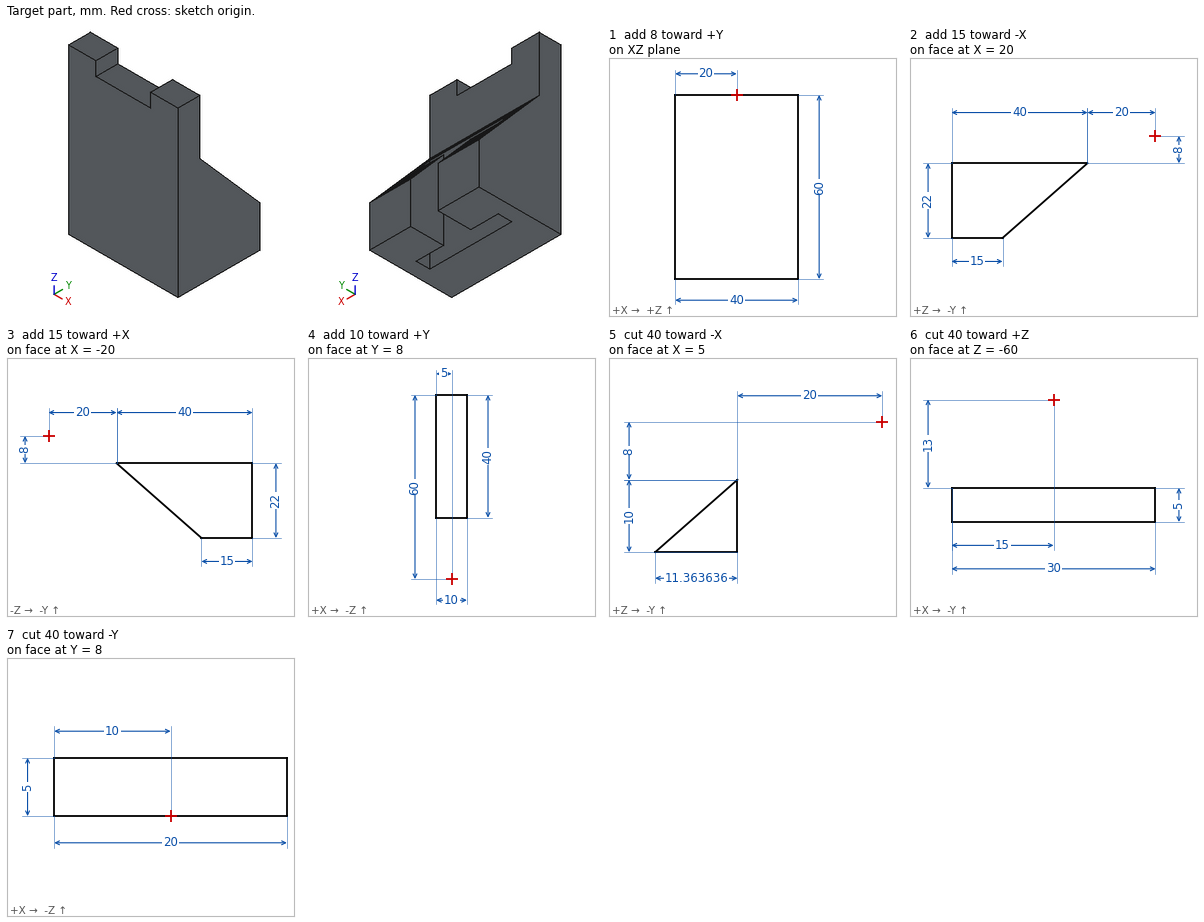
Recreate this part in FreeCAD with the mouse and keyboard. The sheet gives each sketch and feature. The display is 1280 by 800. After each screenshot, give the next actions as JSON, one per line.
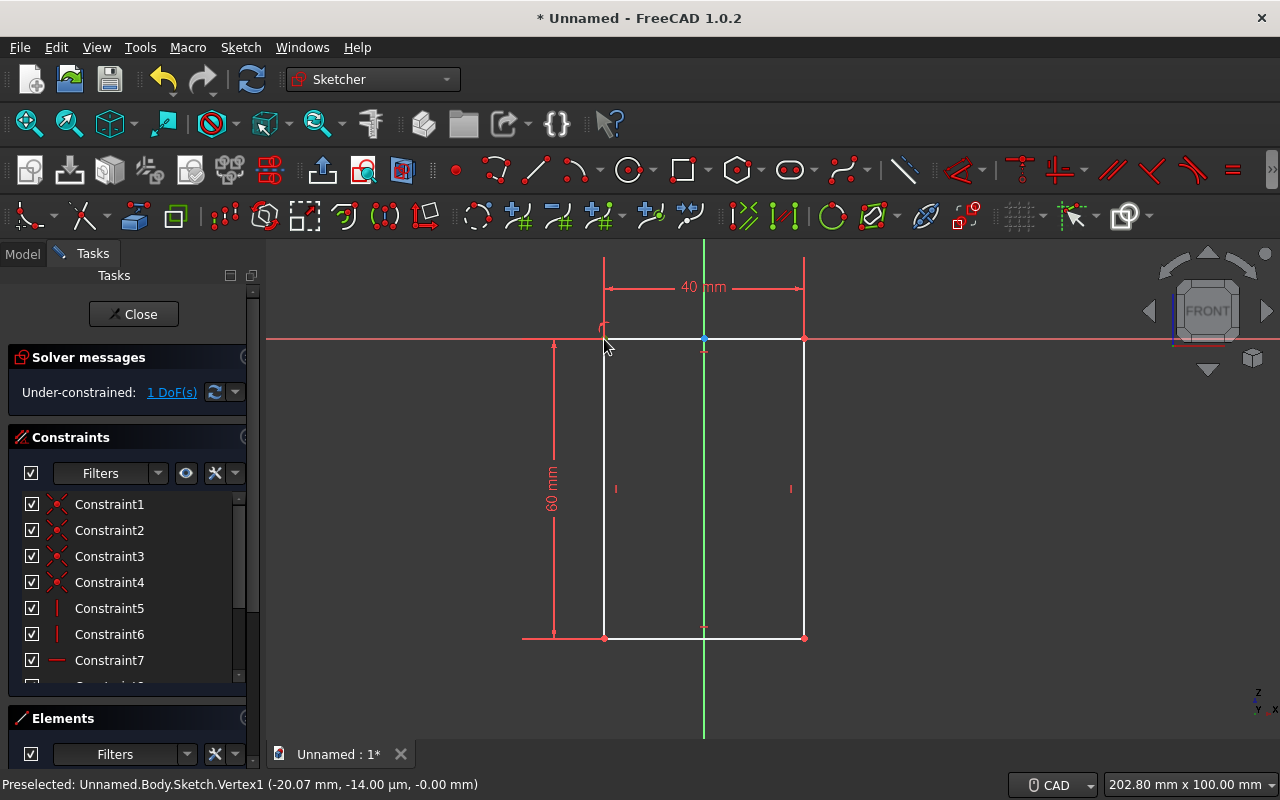
{"action": "key", "text": "l"}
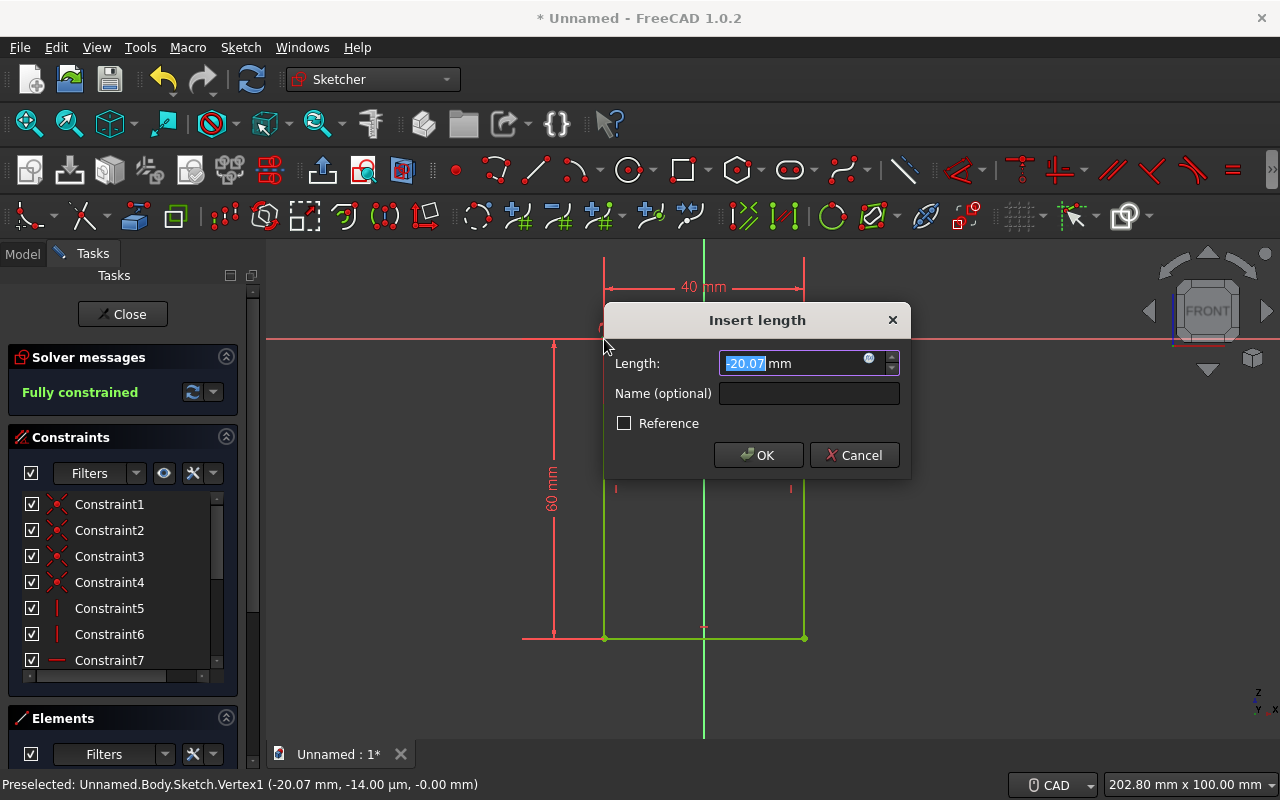
{"action": "type", "text": "-20"}
{"action": "key", "text": "Return"}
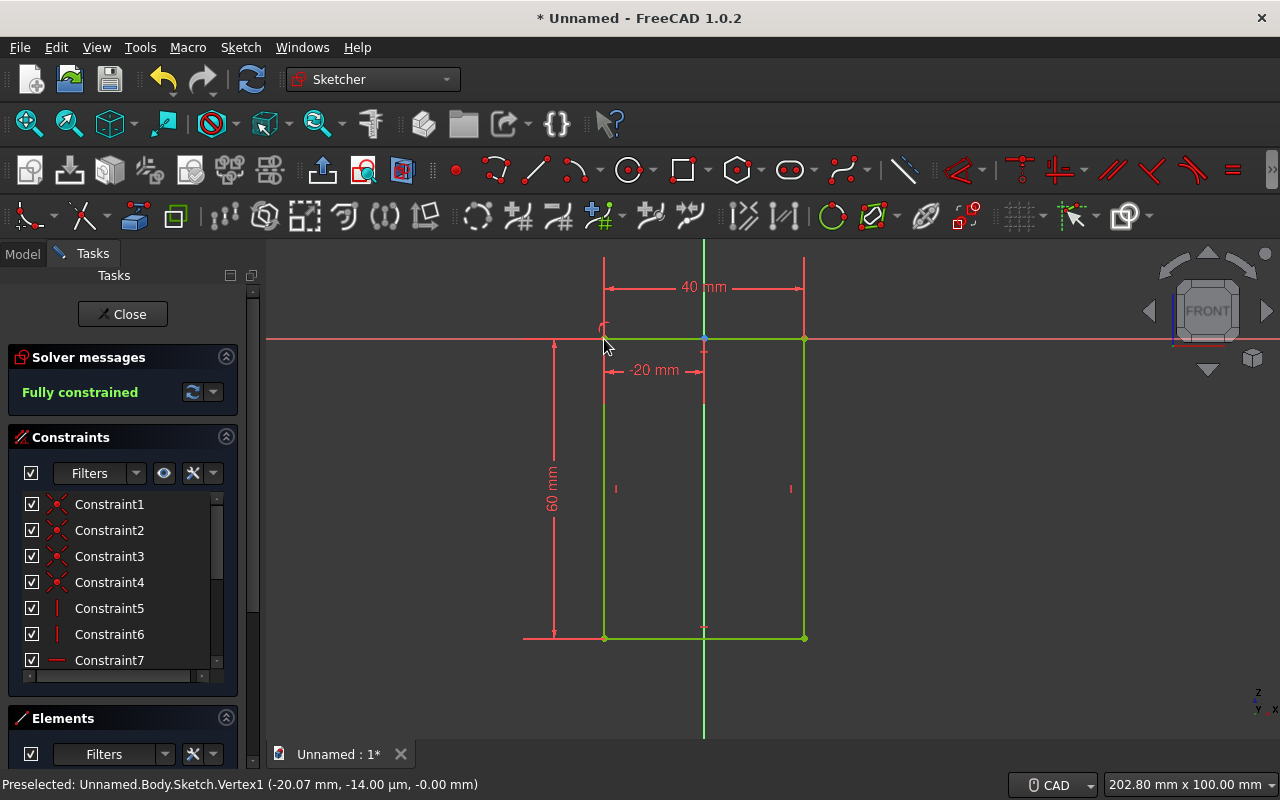
{"action": "left_click", "coordinate": [123, 314]}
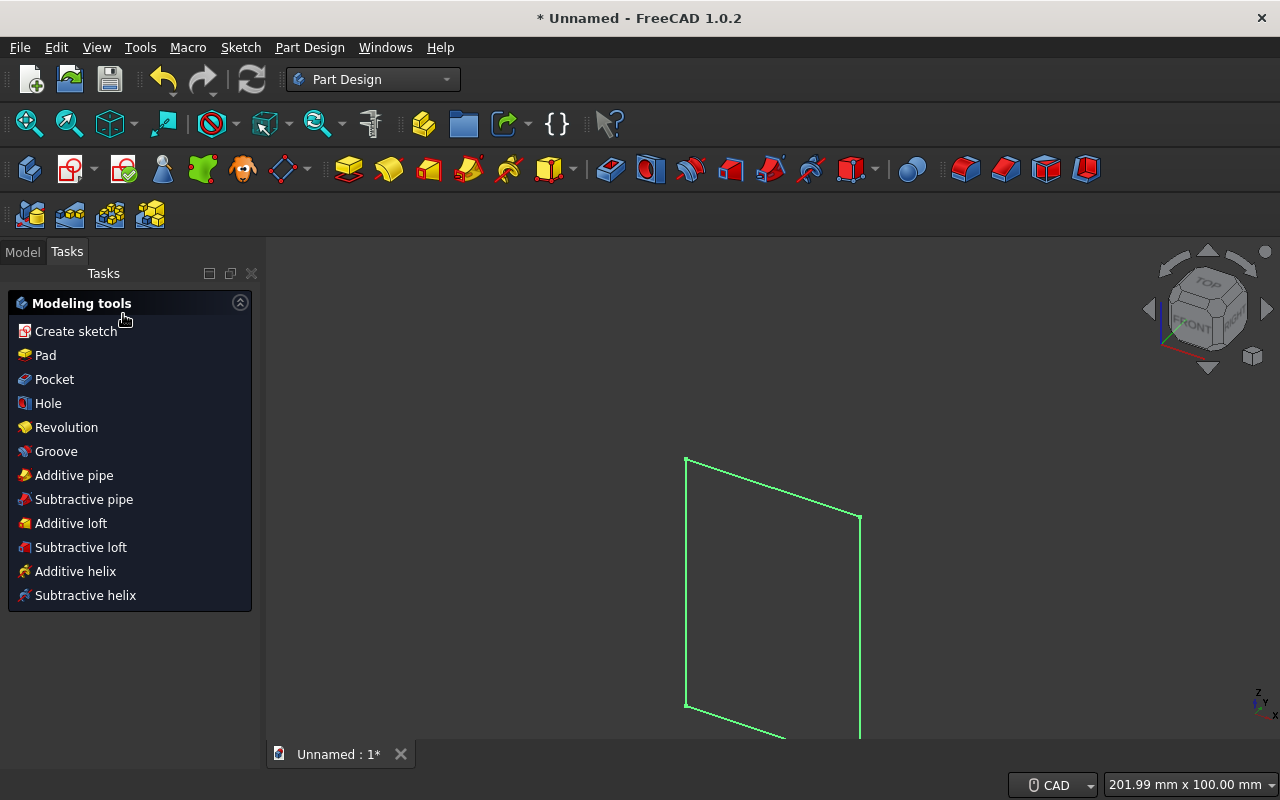
{"action": "left_click", "coordinate": [350, 170]}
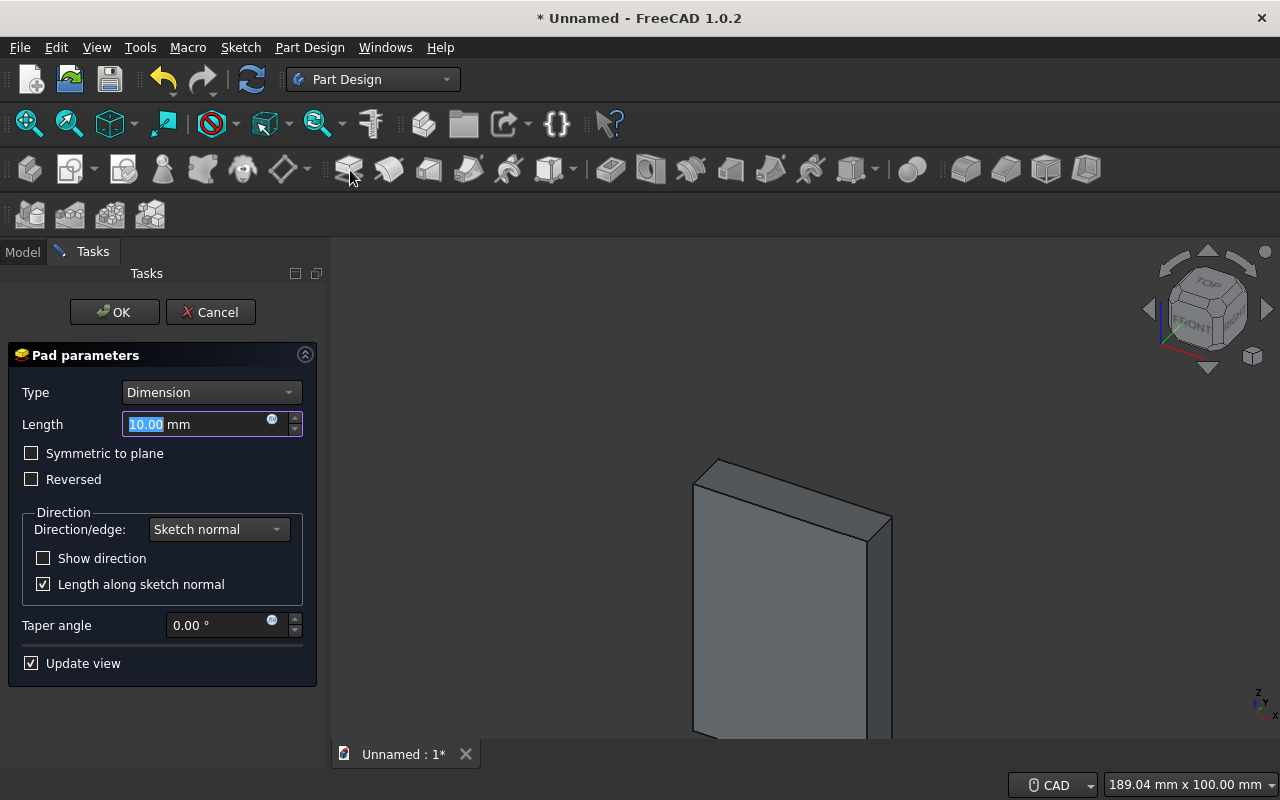
{"action": "type", "text": "8"}
{"action": "key", "text": "Tab"}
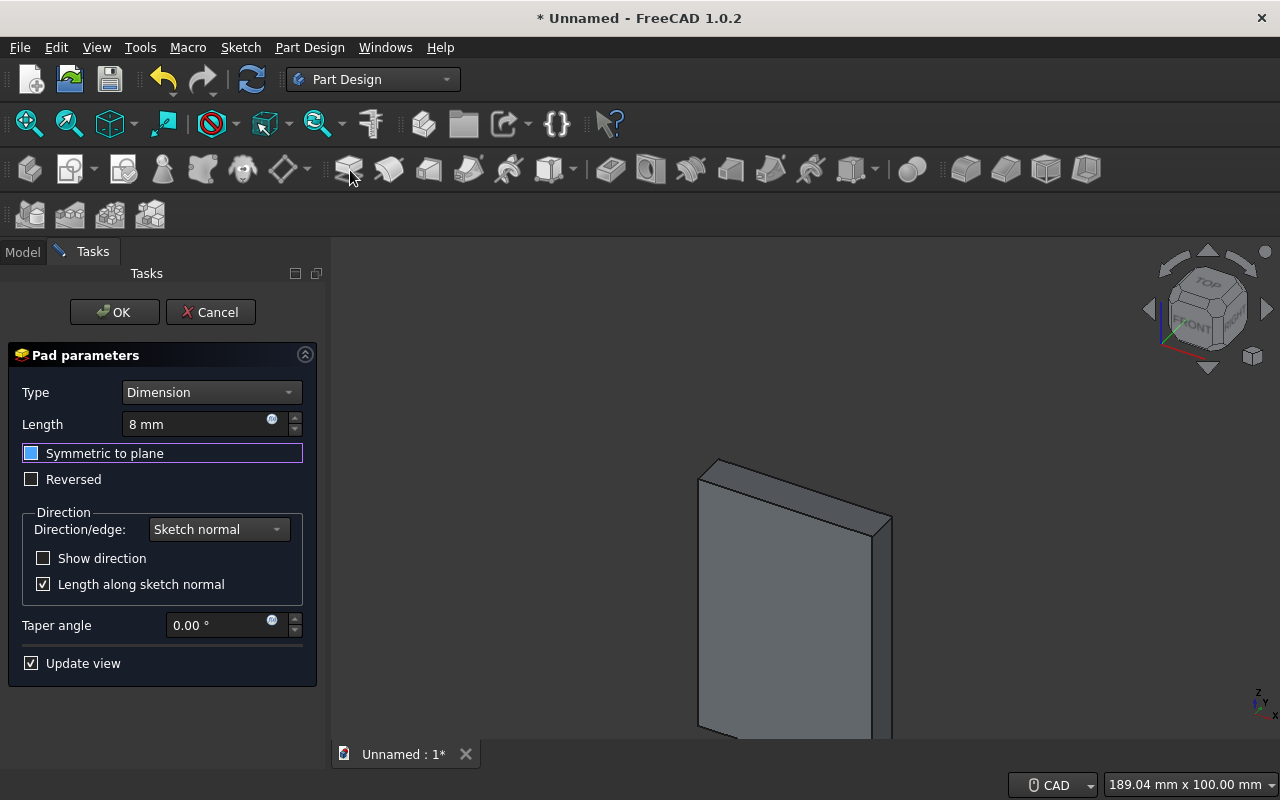
{"action": "left_click", "coordinate": [30, 479]}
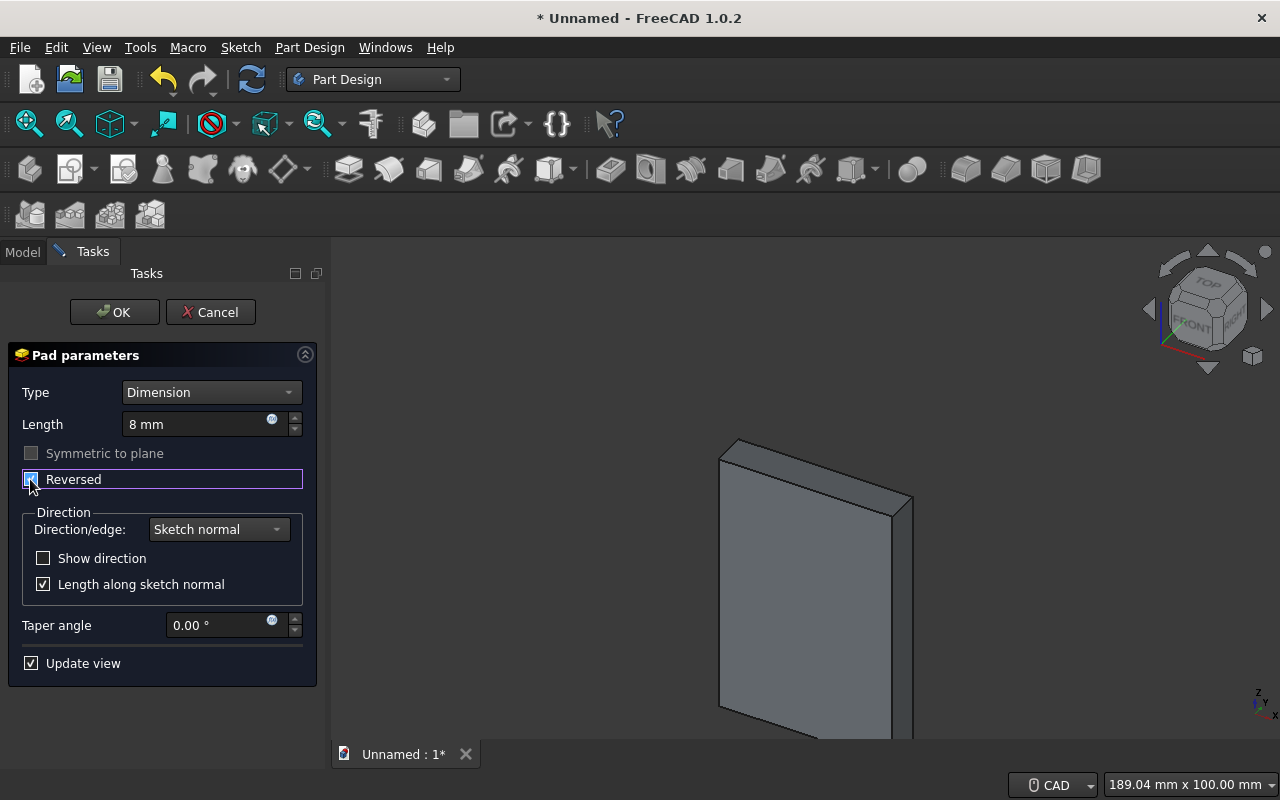
{"action": "left_click", "coordinate": [115, 312]}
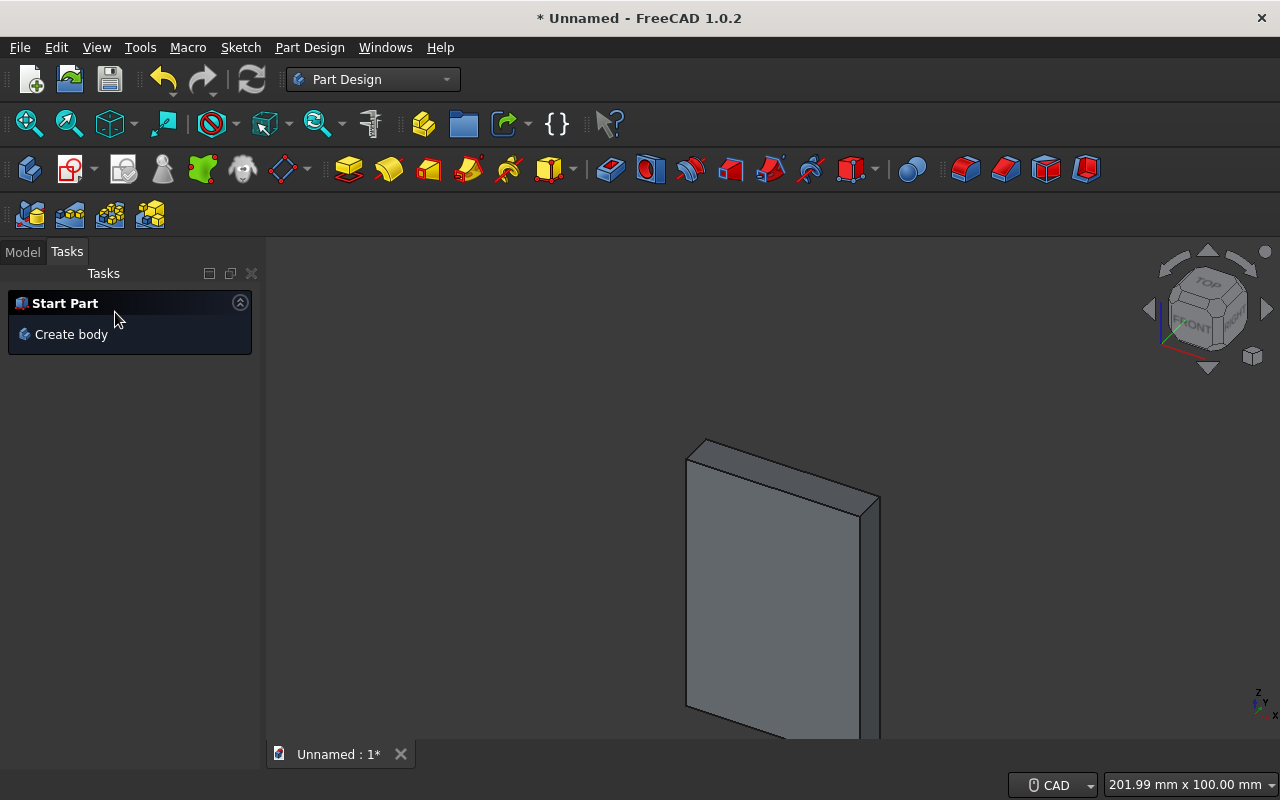
{"action": "left_click", "coordinate": [30, 124]}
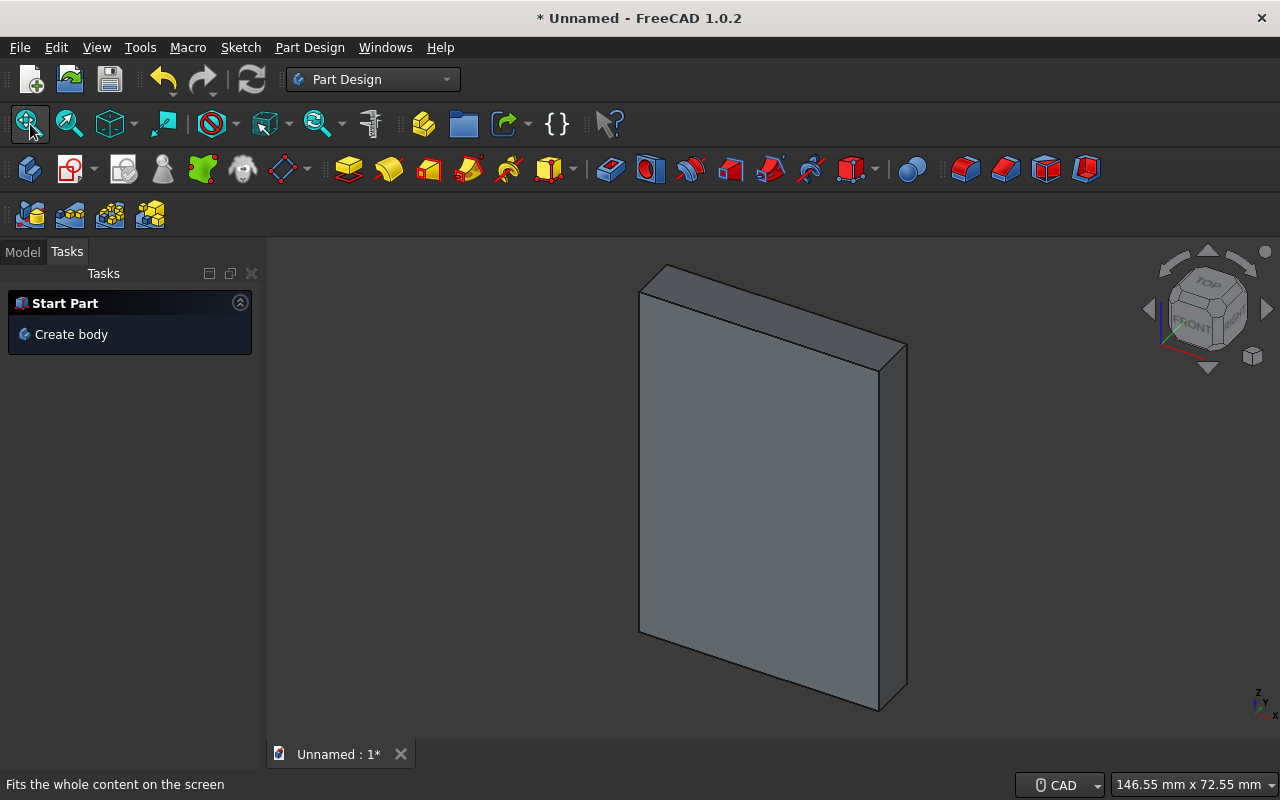
{"action": "left_click", "coordinate": [893, 430]}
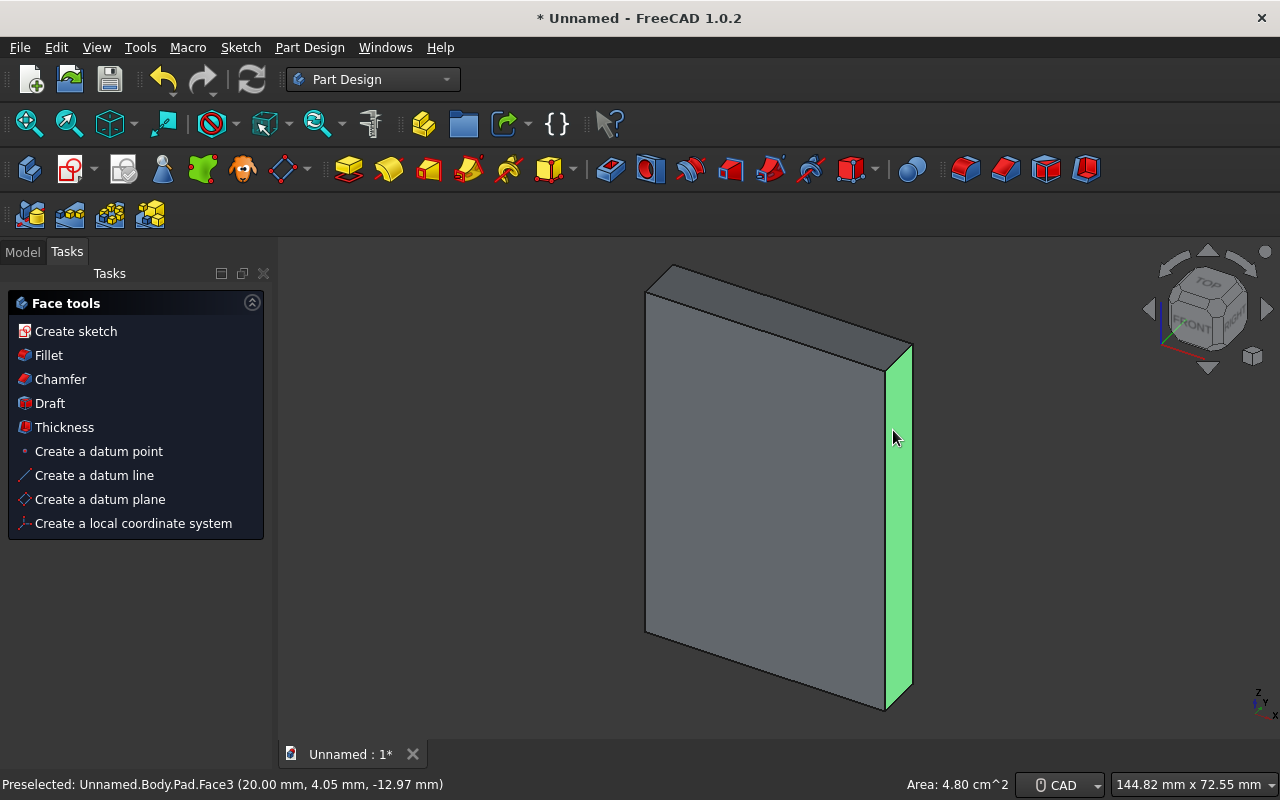
{"action": "left_click", "coordinate": [70, 170]}